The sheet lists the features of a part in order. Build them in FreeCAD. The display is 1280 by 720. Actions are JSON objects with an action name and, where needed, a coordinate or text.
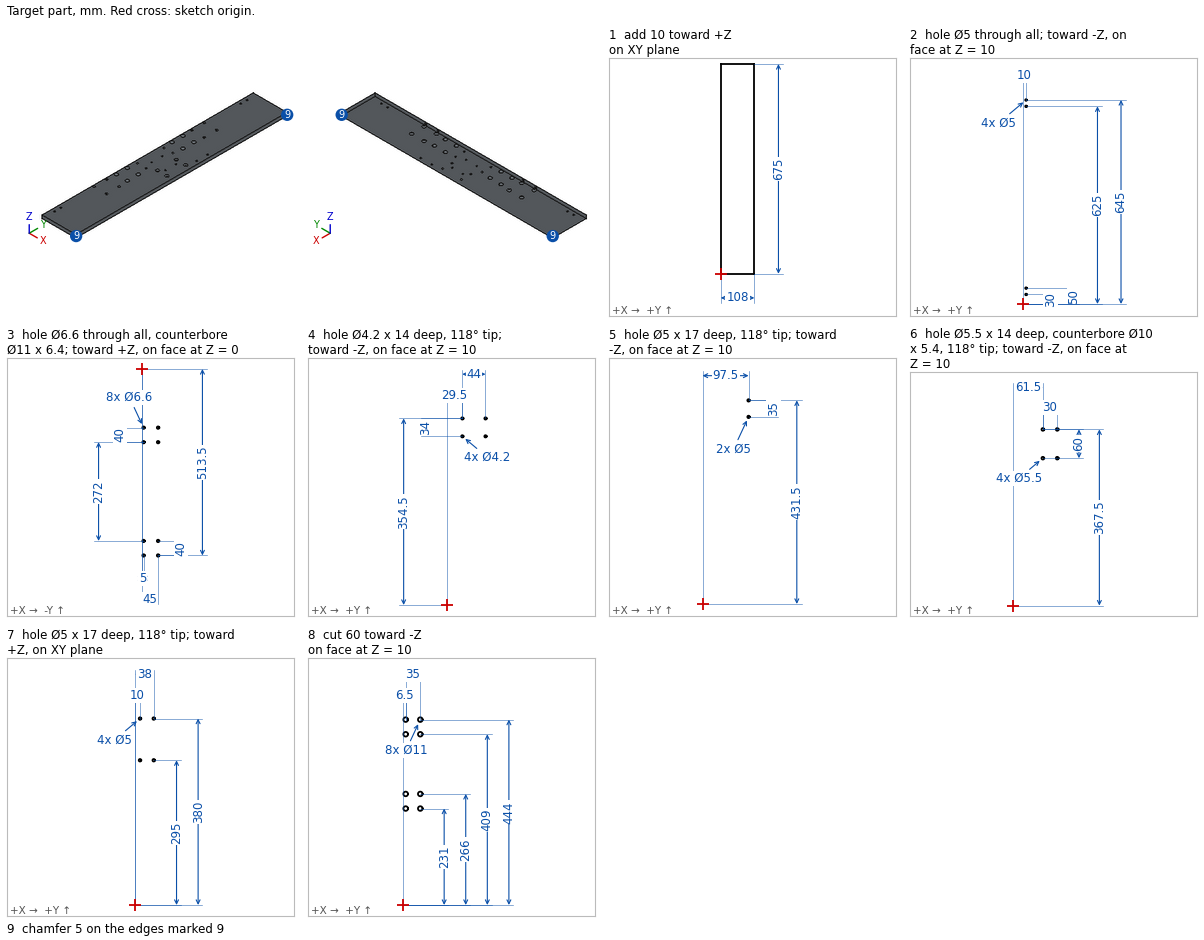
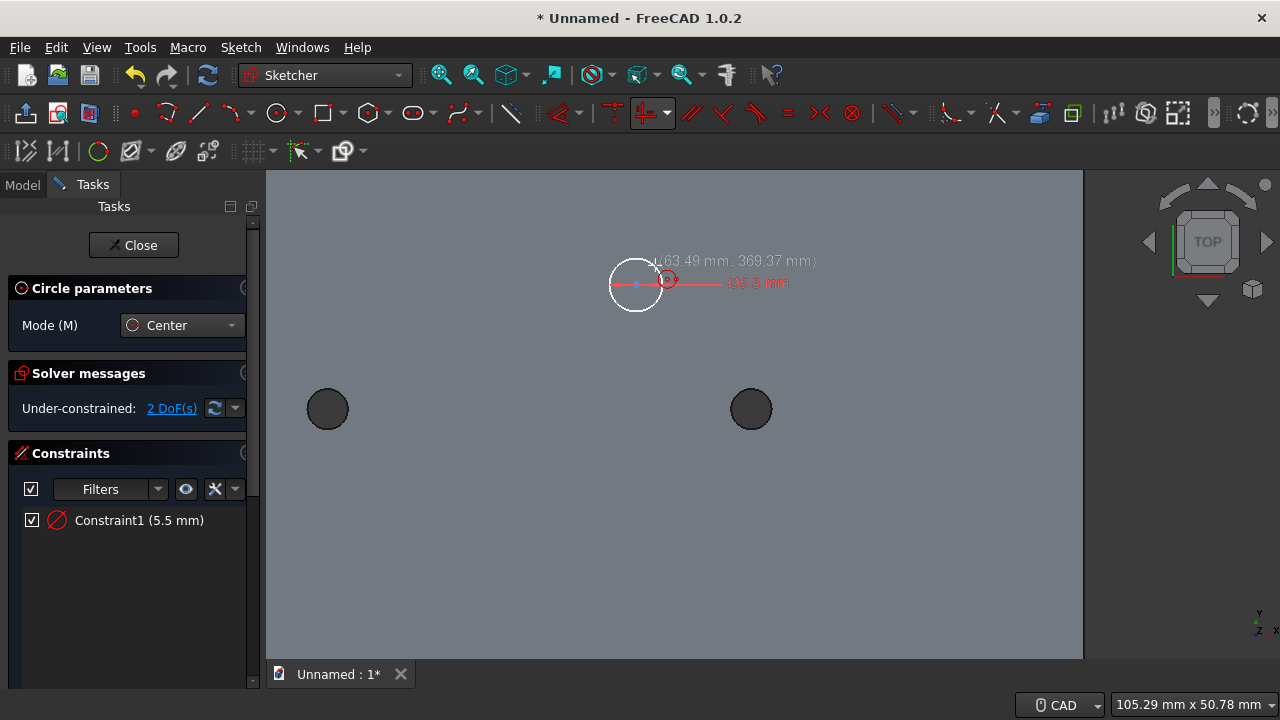
{"action": "left_click", "coordinate": [925, 284]}
{"action": "mouse_move", "coordinate": [943, 265]}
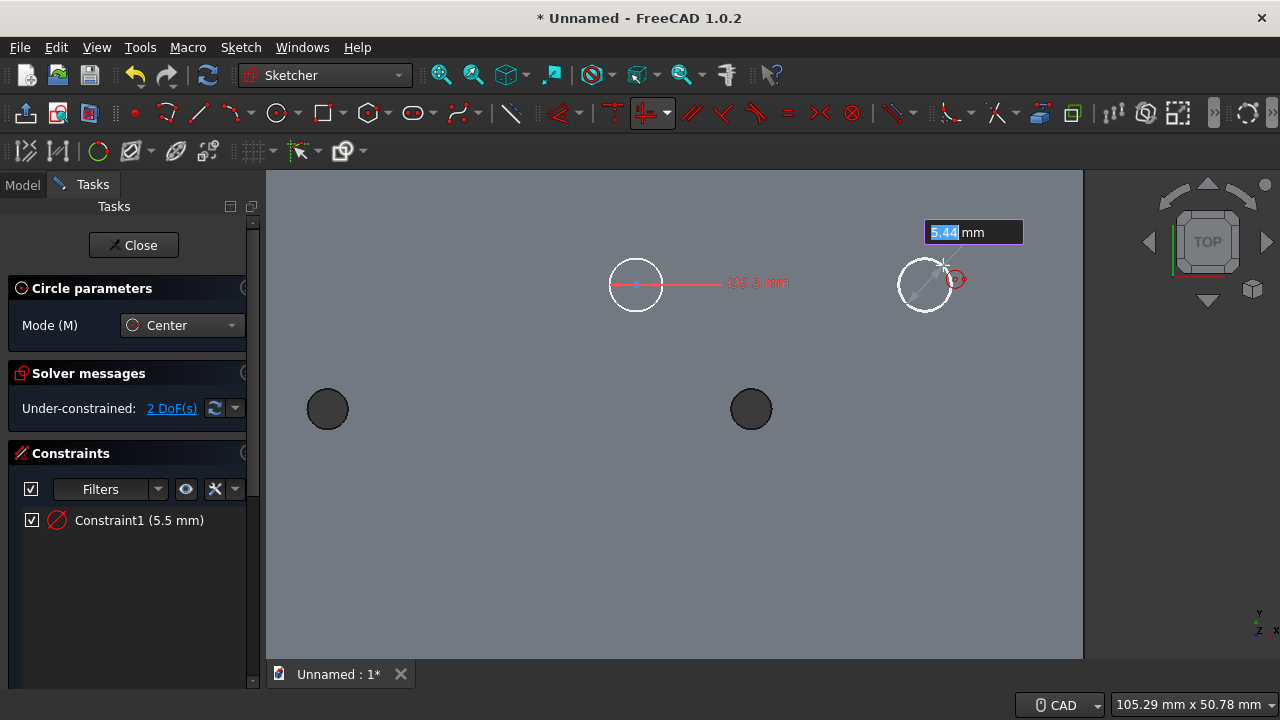
{"action": "type", "text": "5.5"}
{"action": "key", "text": "Return"}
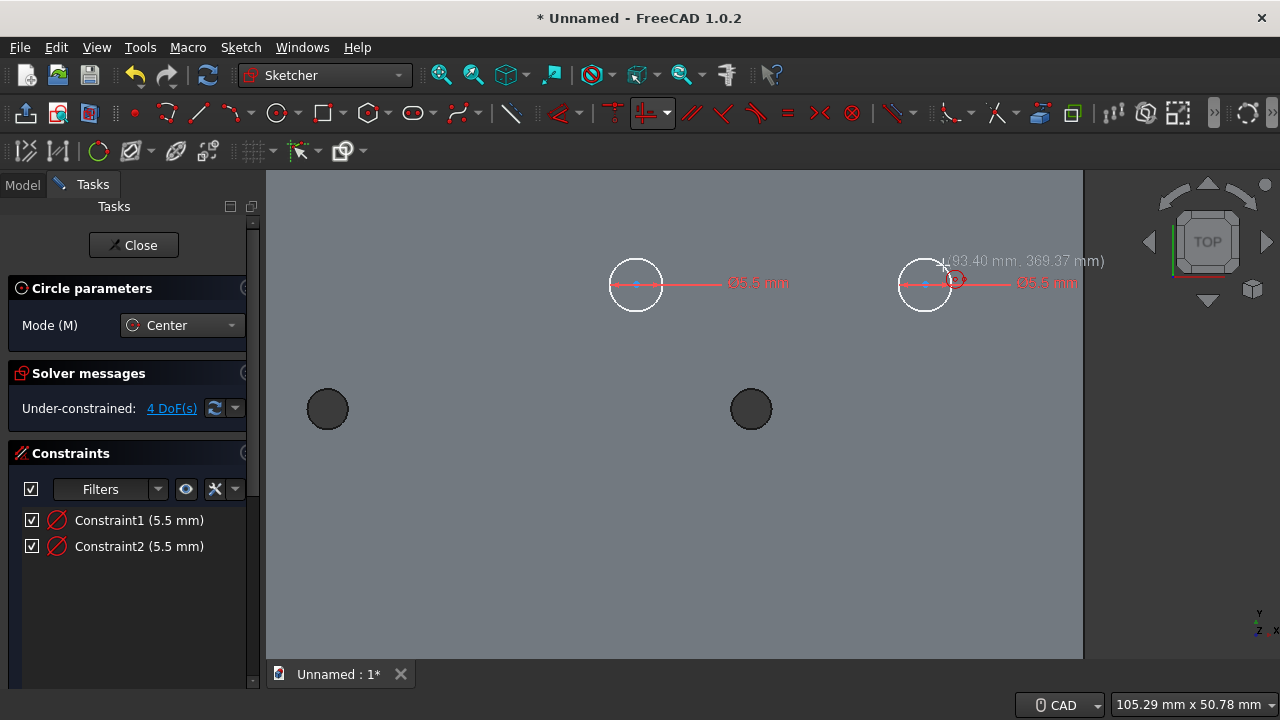
{"action": "scroll", "coordinate": [643, 285], "scroll_direction": "down", "scroll_amount": 4}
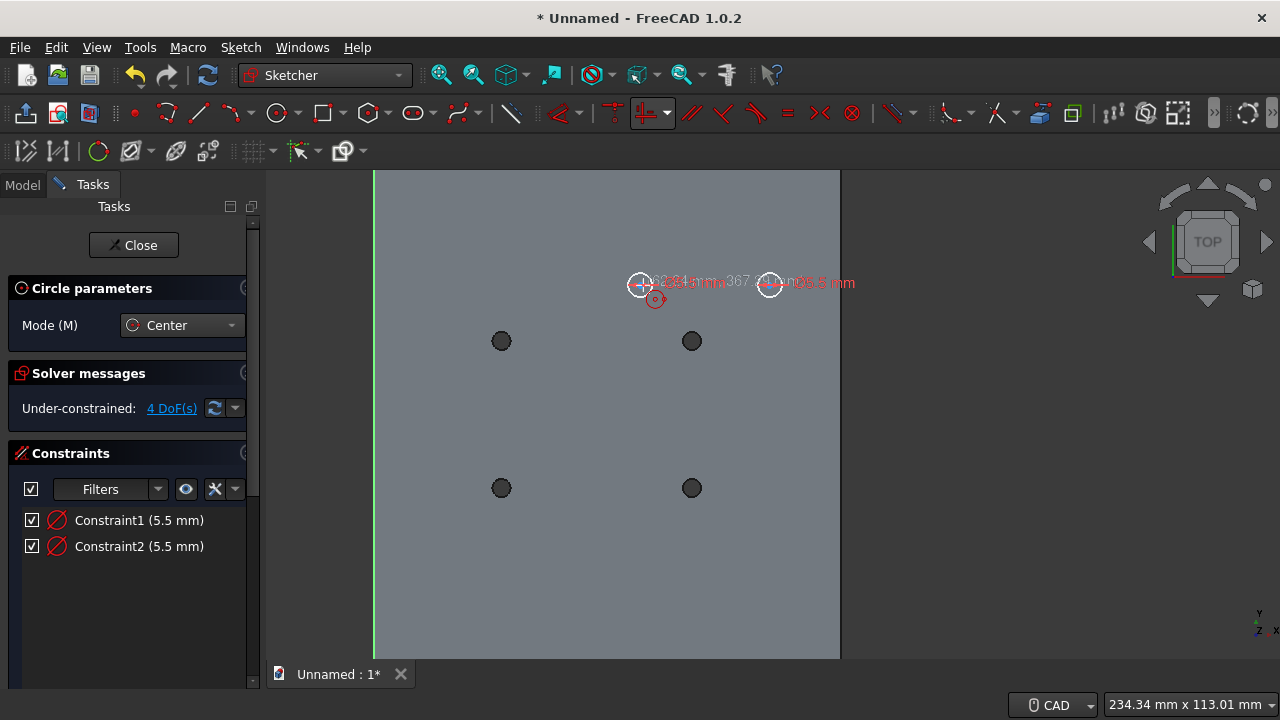
{"action": "scroll", "coordinate": [640, 544], "scroll_direction": "up", "scroll_amount": 4}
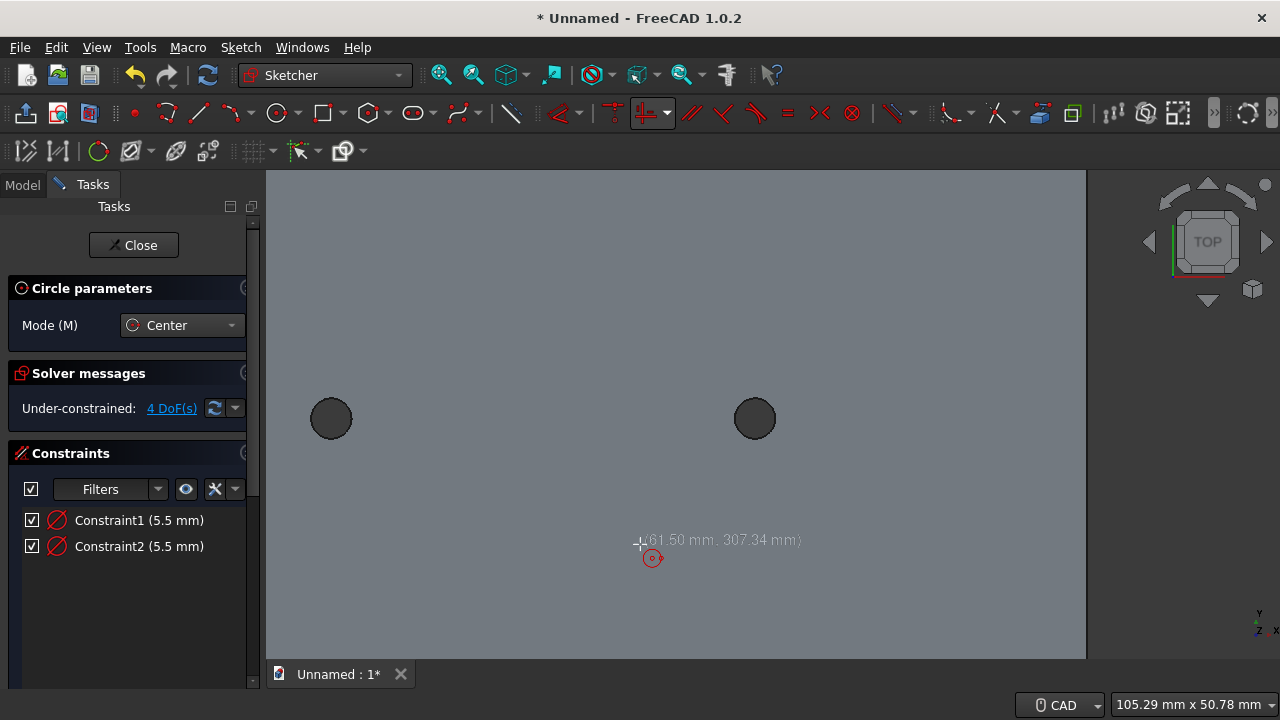
{"action": "left_click", "coordinate": [640, 544]}
{"action": "mouse_move", "coordinate": [658, 525]}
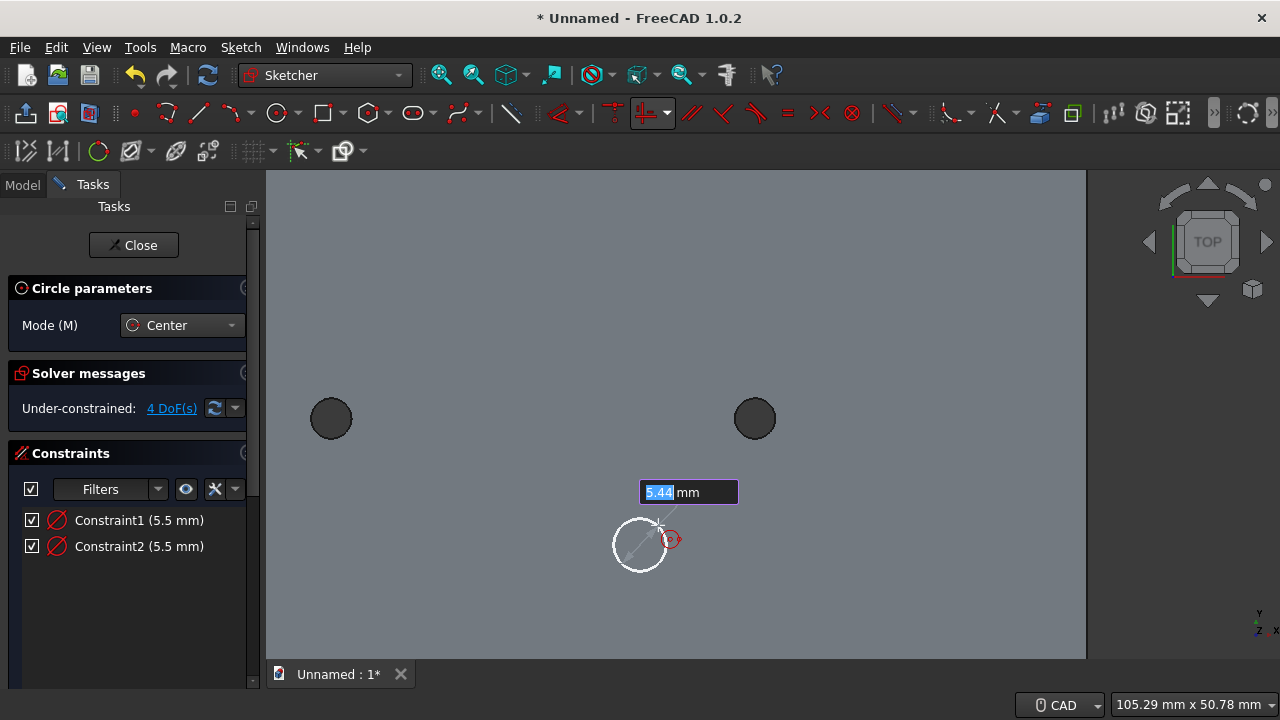
{"action": "type", "text": "5.5"}
{"action": "key", "text": "Return"}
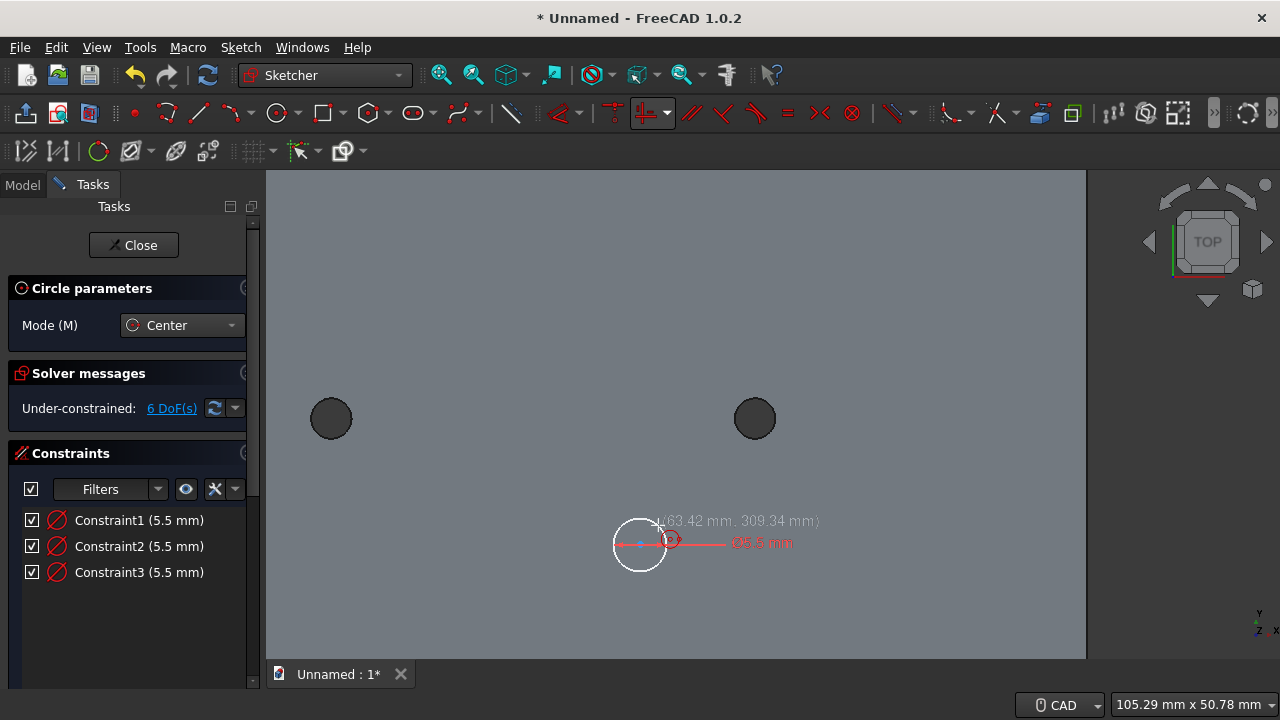
{"action": "left_click", "coordinate": [928, 544]}
{"action": "mouse_move", "coordinate": [947, 525]}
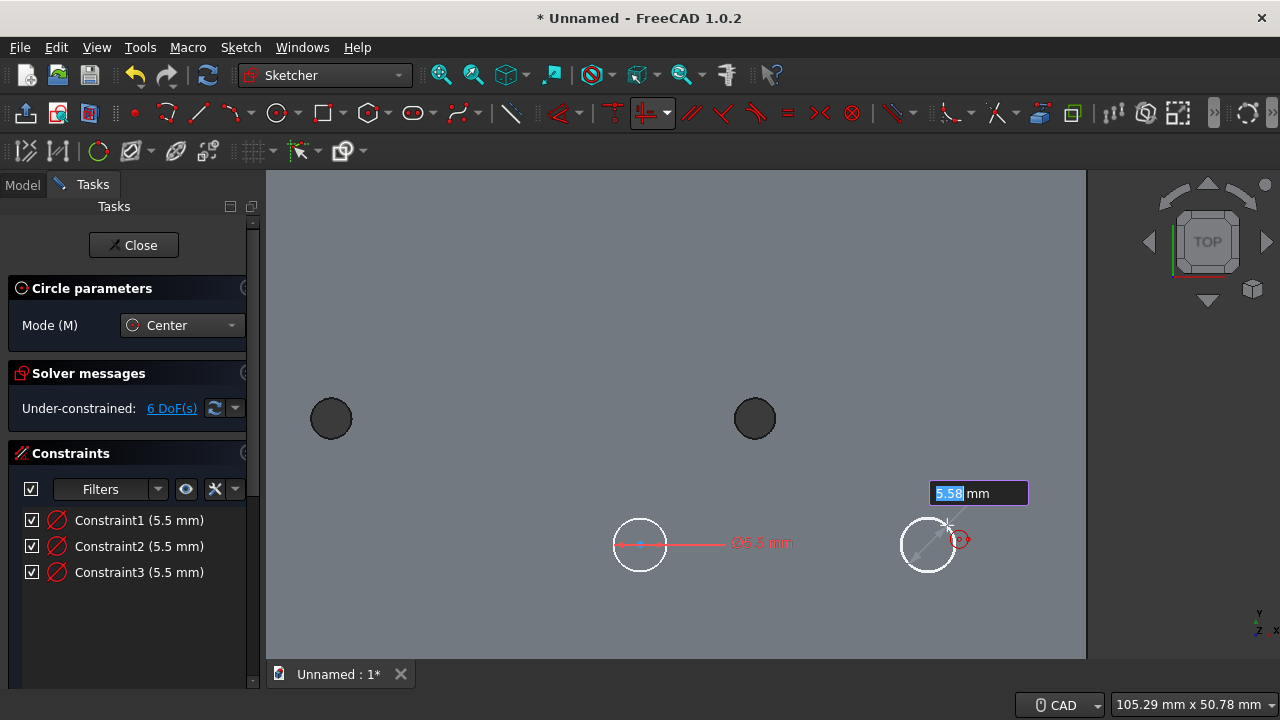
{"action": "type", "text": "5.5"}
{"action": "key", "text": "Return"}
{"action": "key", "text": "Escape"}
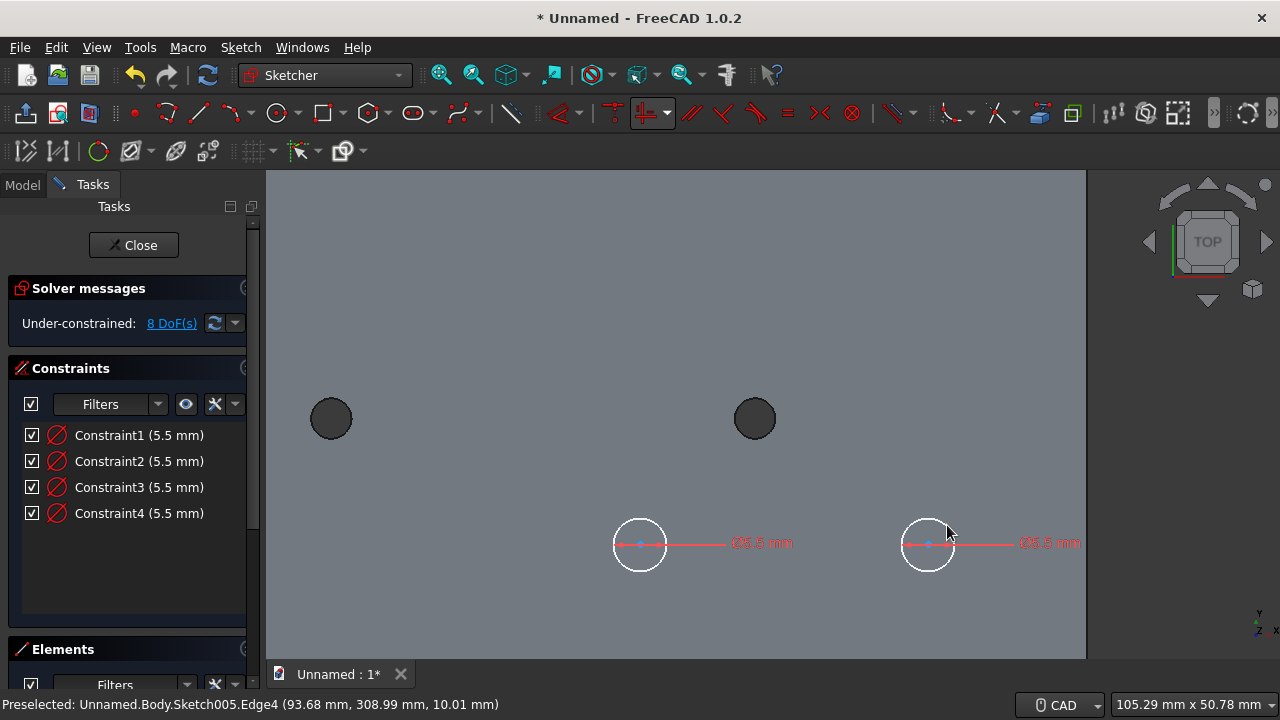
{"action": "scroll", "coordinate": [640, 545], "scroll_direction": "down", "scroll_amount": 4}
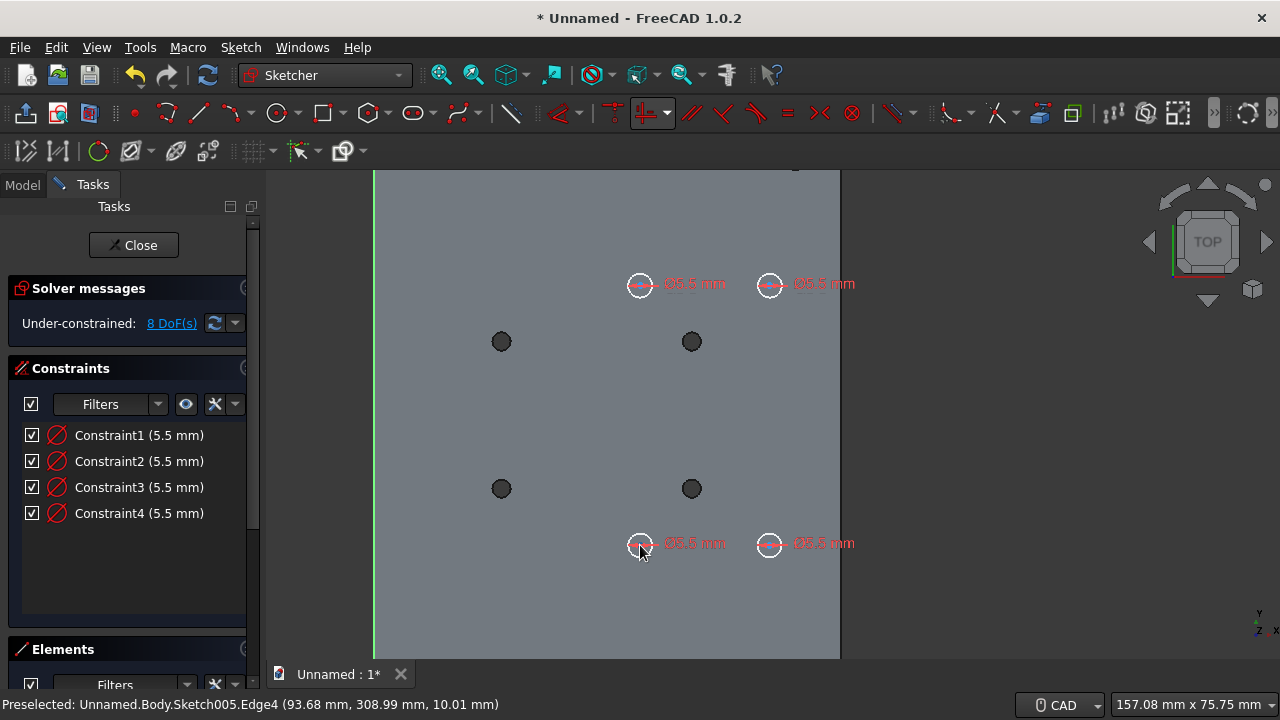
{"action": "left_click", "coordinate": [640, 286]}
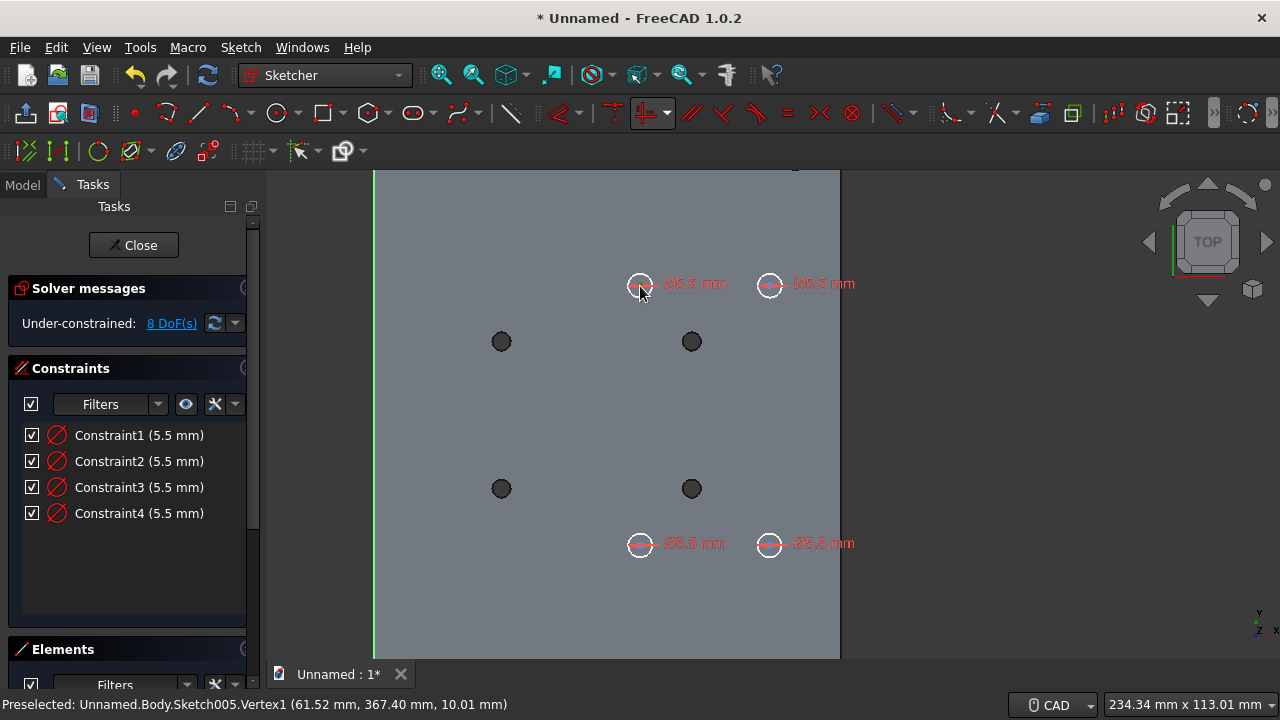
{"action": "left_click", "coordinate": [770, 286]}